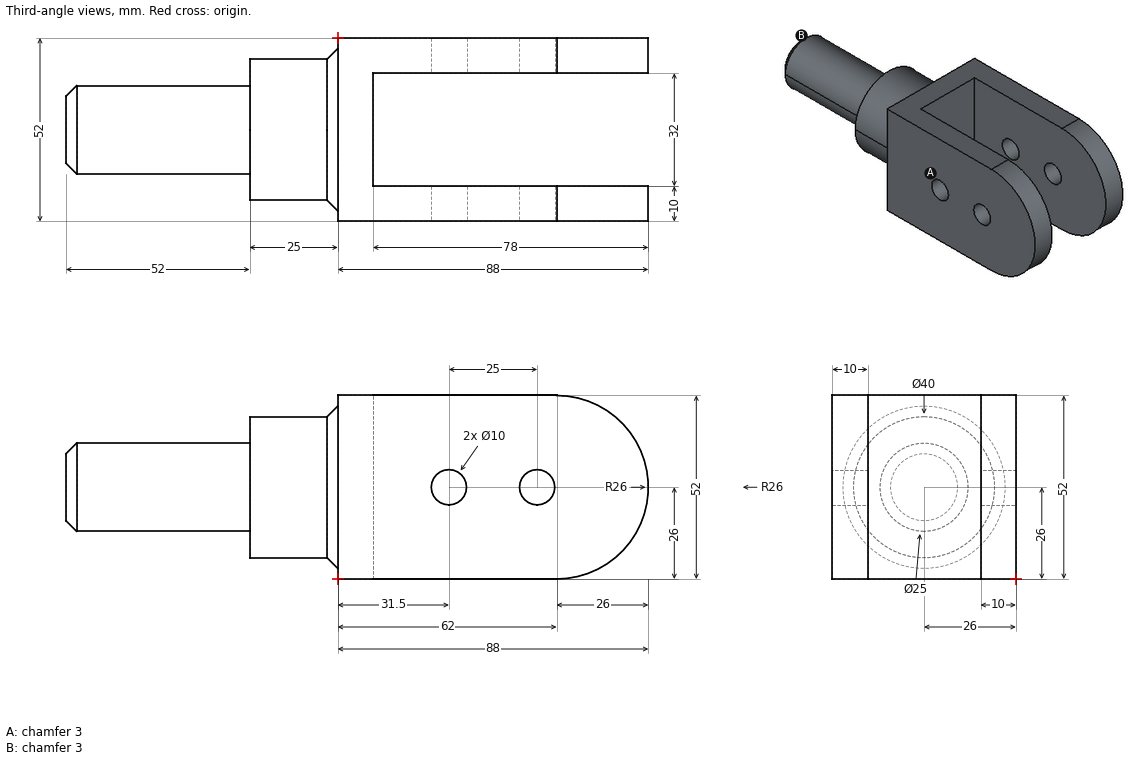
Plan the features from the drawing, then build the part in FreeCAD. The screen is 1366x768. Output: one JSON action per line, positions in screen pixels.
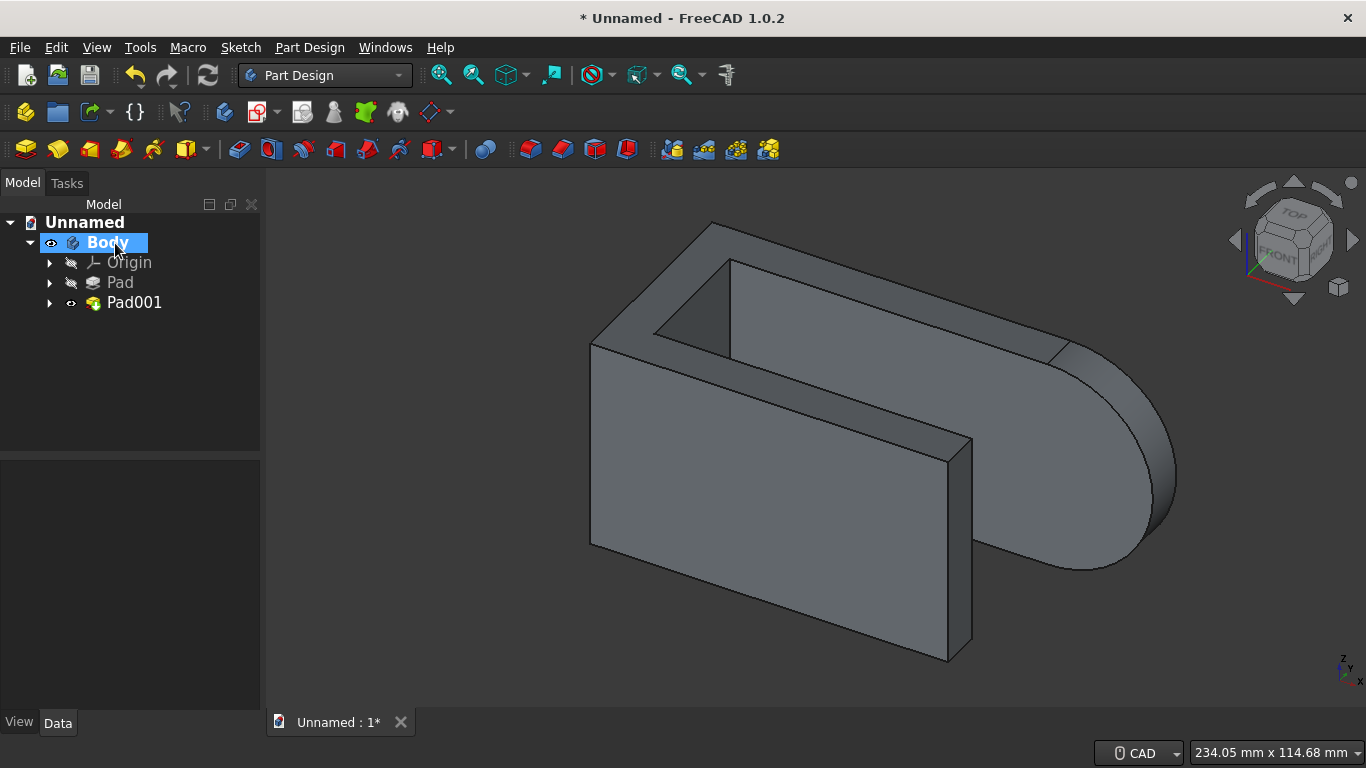
{"action": "left_click", "coordinate": [50, 263]}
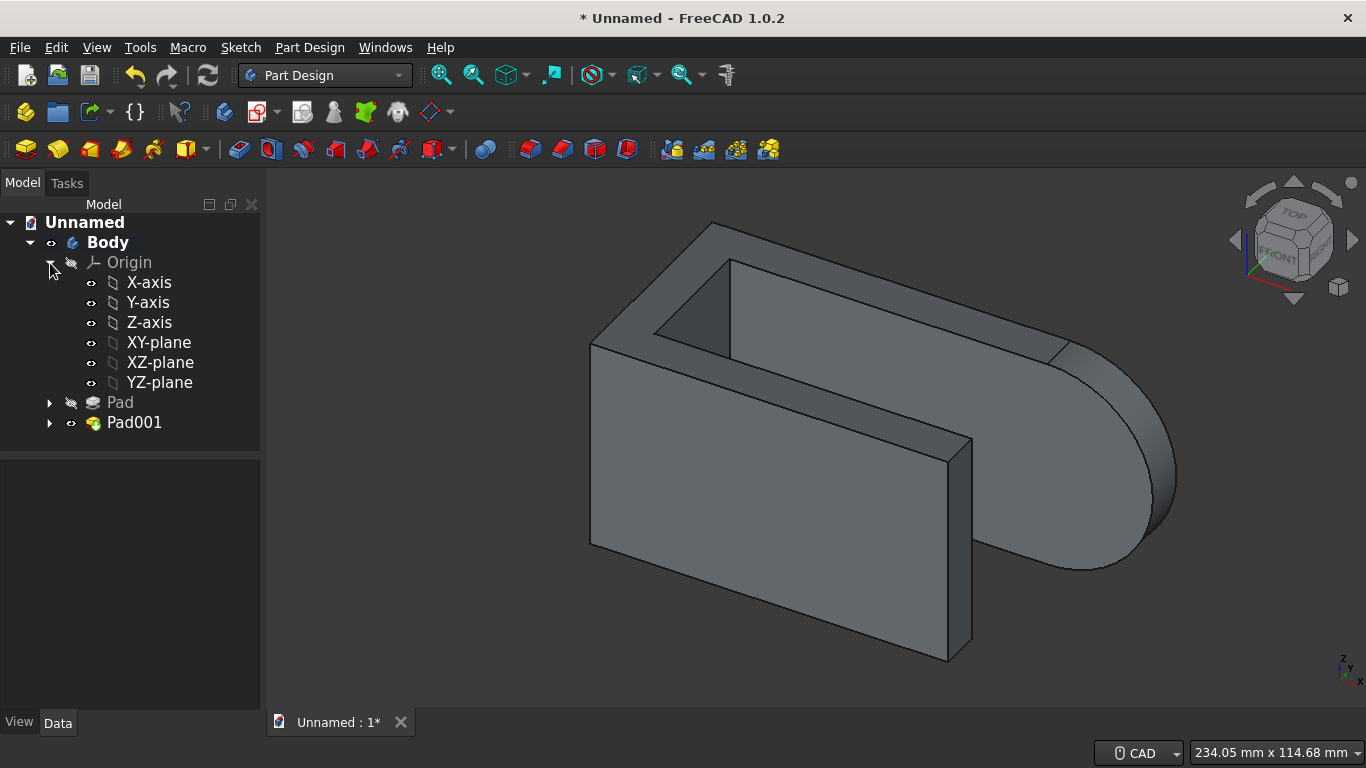
{"action": "left_click", "coordinate": [136, 363]}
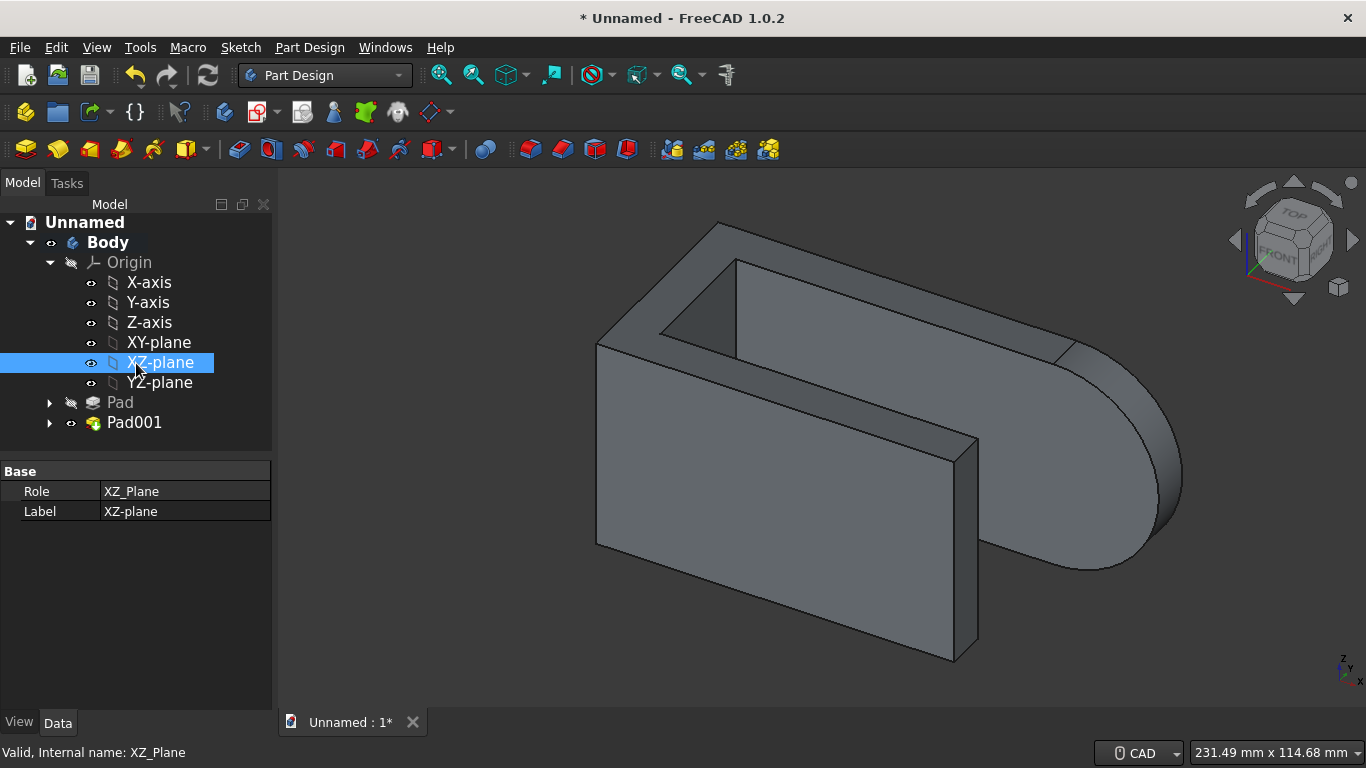
{"action": "left_click", "coordinate": [430, 112]}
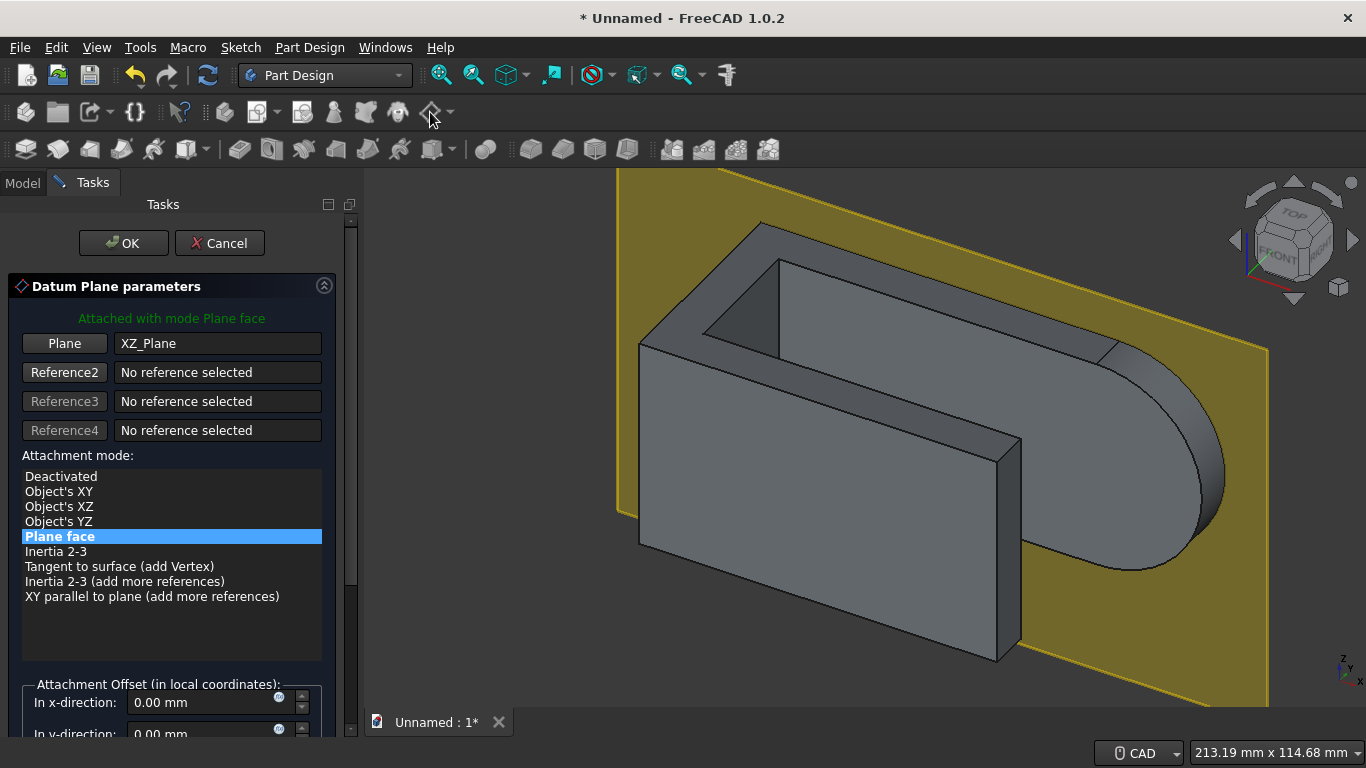
{"action": "scroll", "coordinate": [351, 475], "scroll_direction": "down", "scroll_amount": 2}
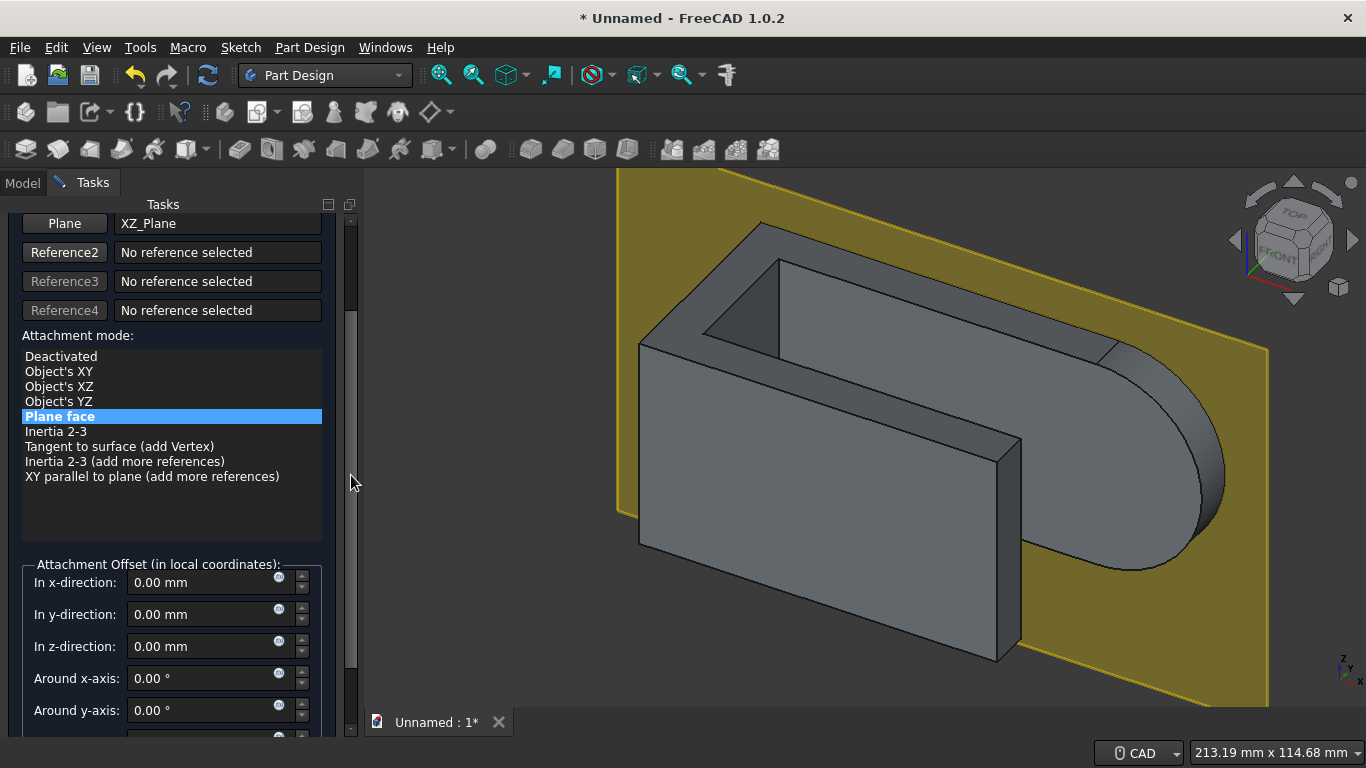
{"action": "triple_click", "coordinate": [210, 646]}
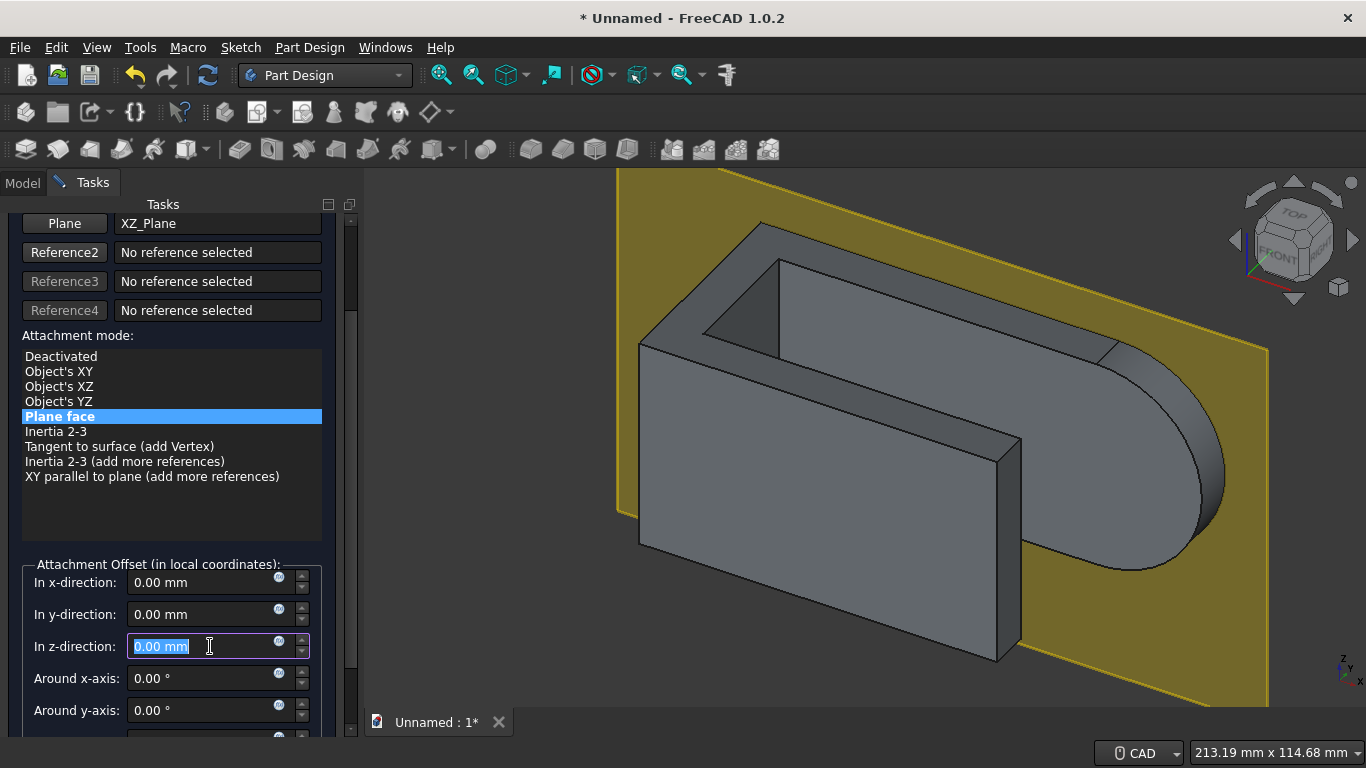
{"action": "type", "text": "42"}
{"action": "key", "text": "Tab"}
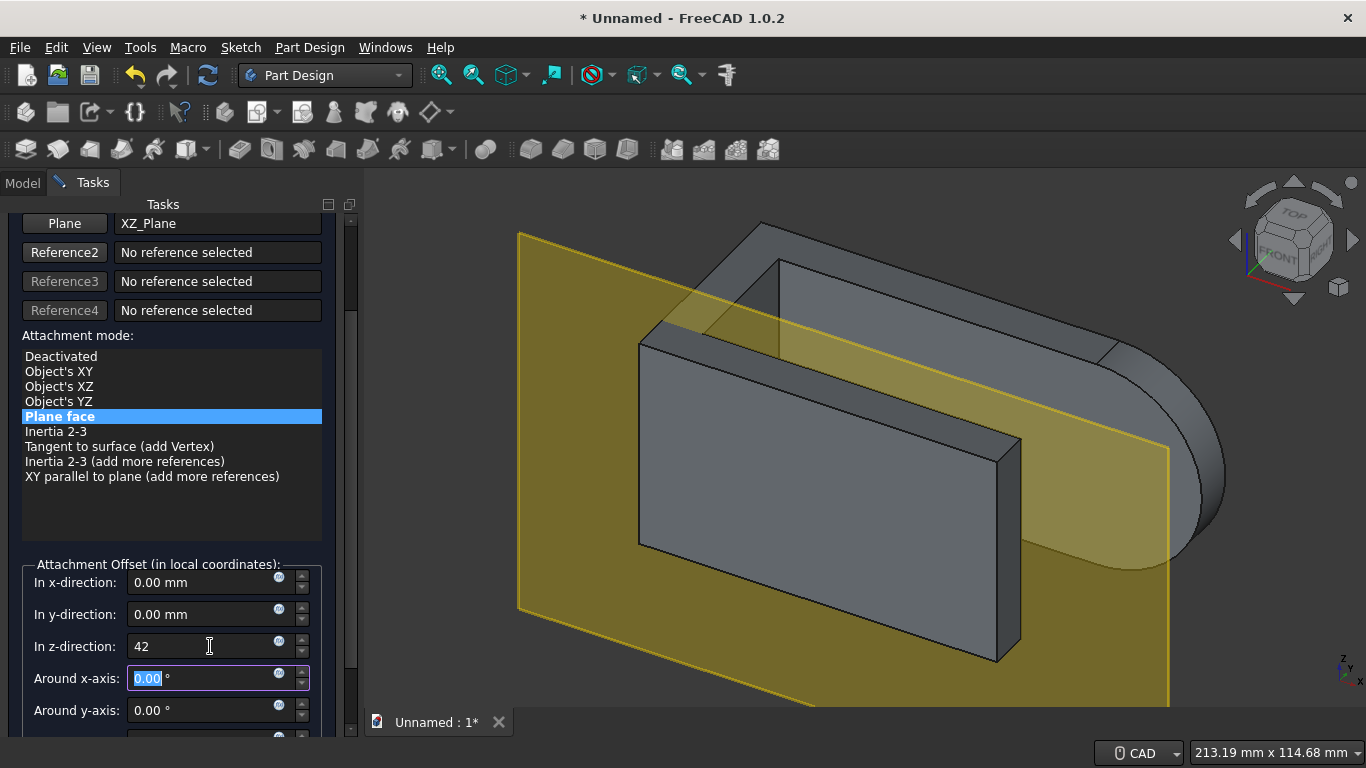
{"action": "scroll", "coordinate": [351, 475], "scroll_direction": "up", "scroll_amount": 3}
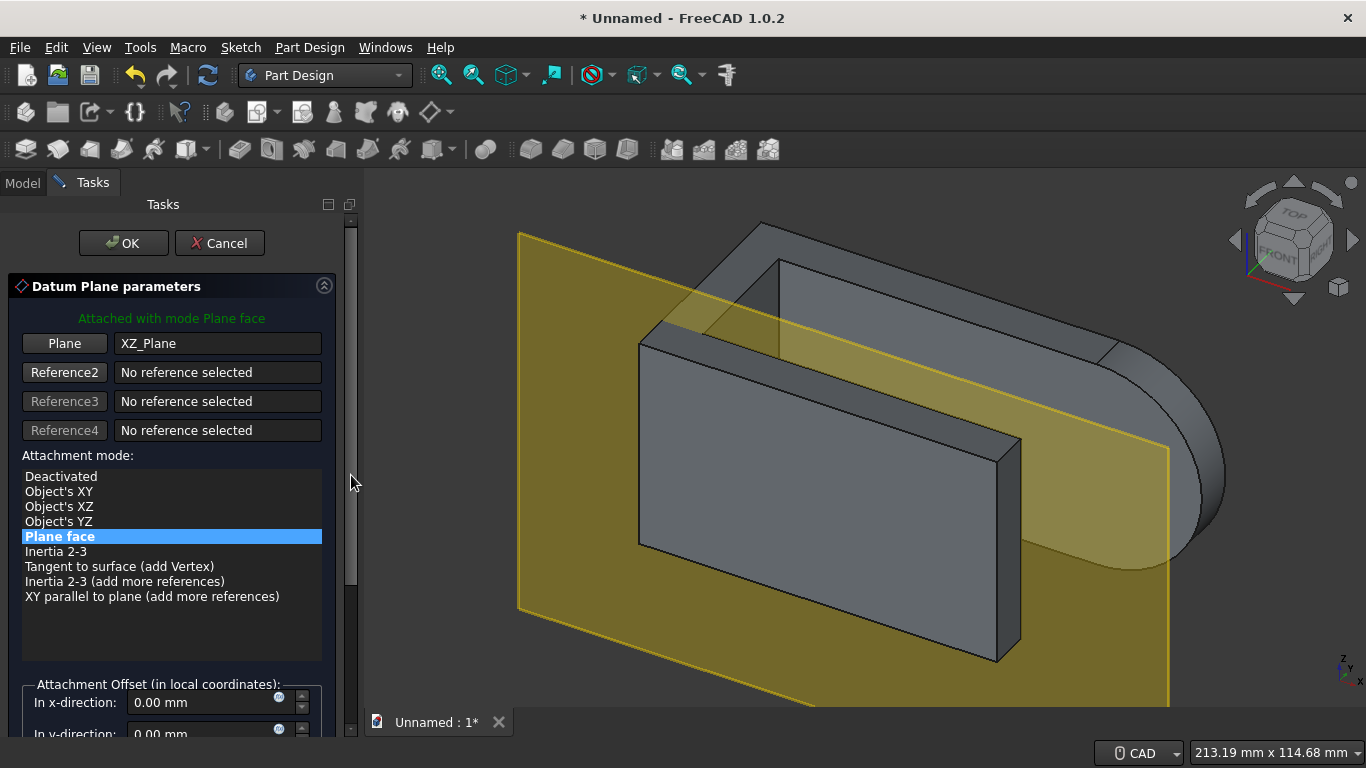
{"action": "left_click", "coordinate": [124, 243]}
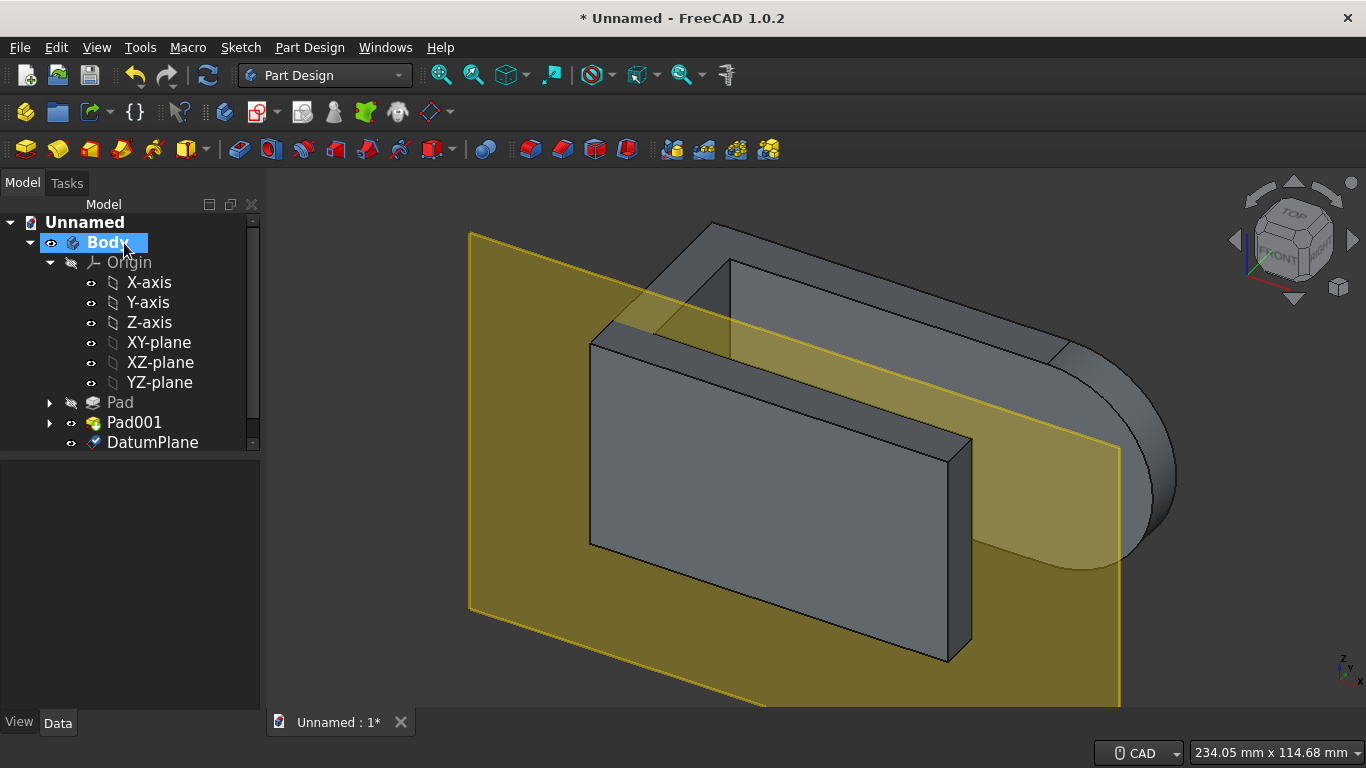
{"action": "left_click", "coordinate": [116, 443]}